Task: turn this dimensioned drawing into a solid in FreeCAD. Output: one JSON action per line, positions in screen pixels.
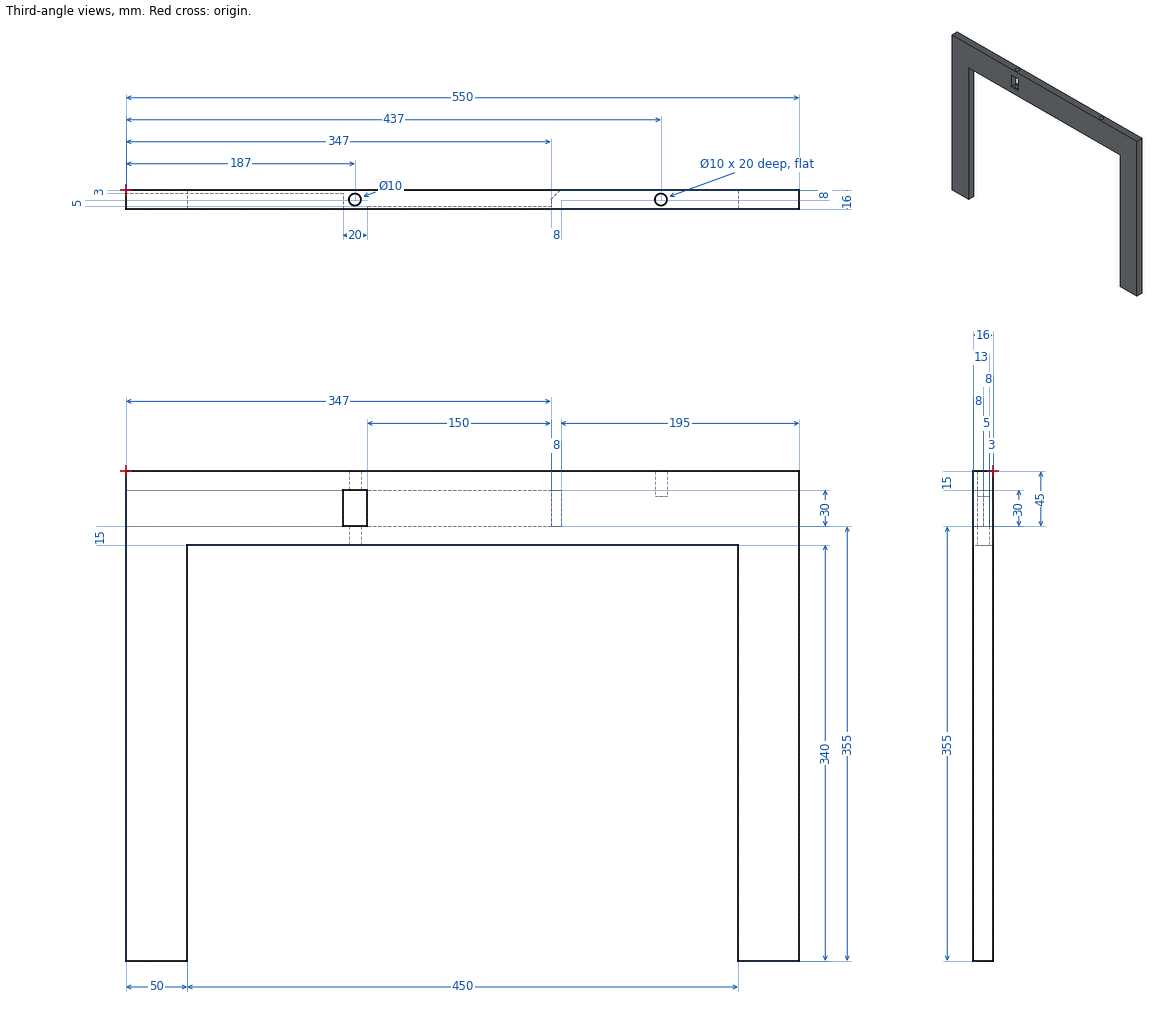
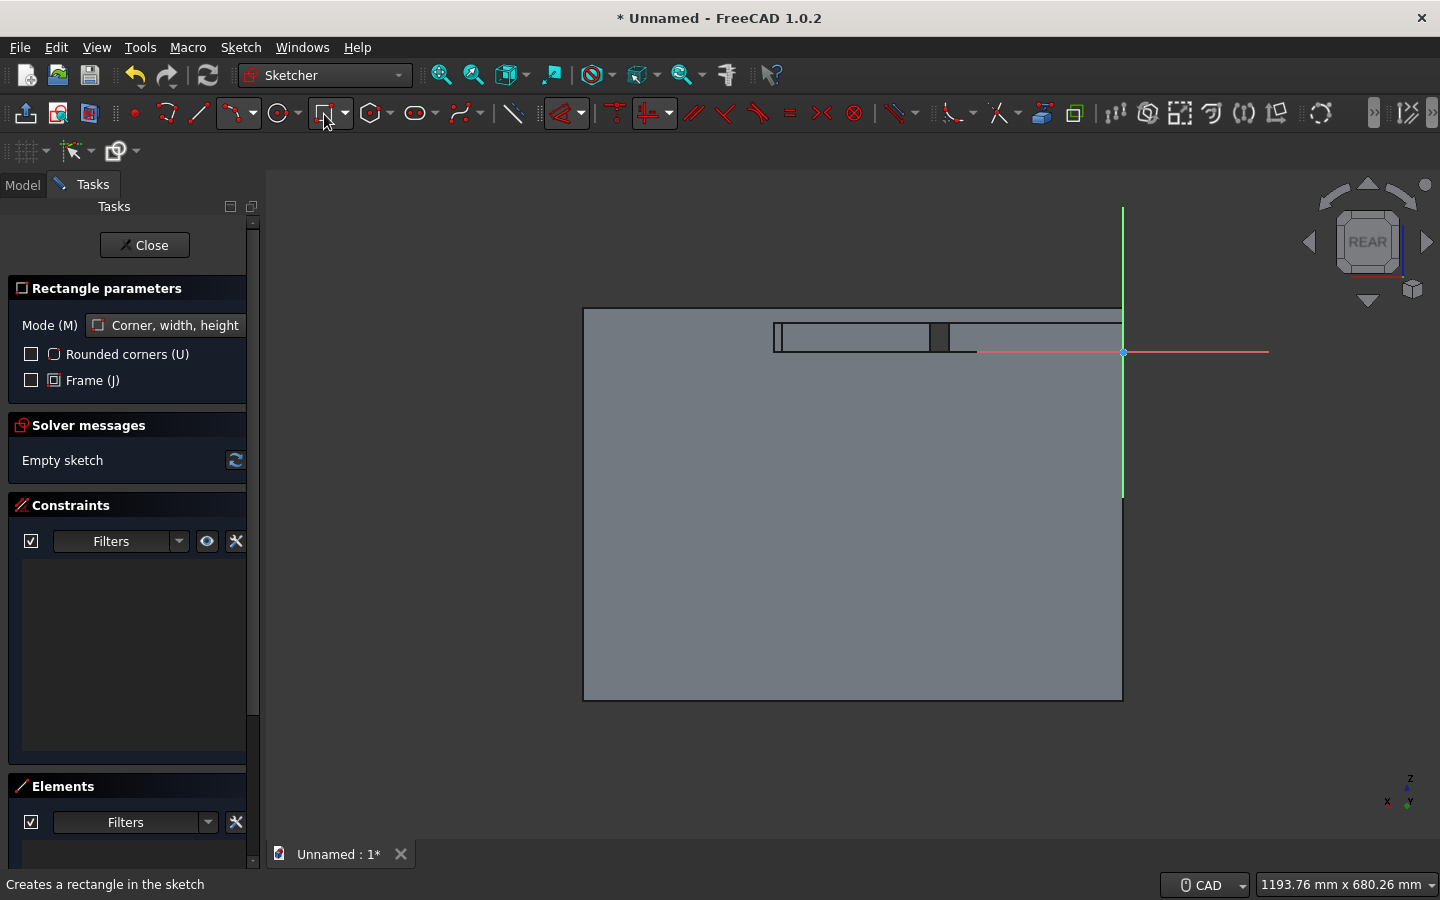
{"action": "left_click", "coordinate": [632, 367]}
{"action": "left_click", "coordinate": [1074, 701]}
{"action": "key", "text": "Escape"}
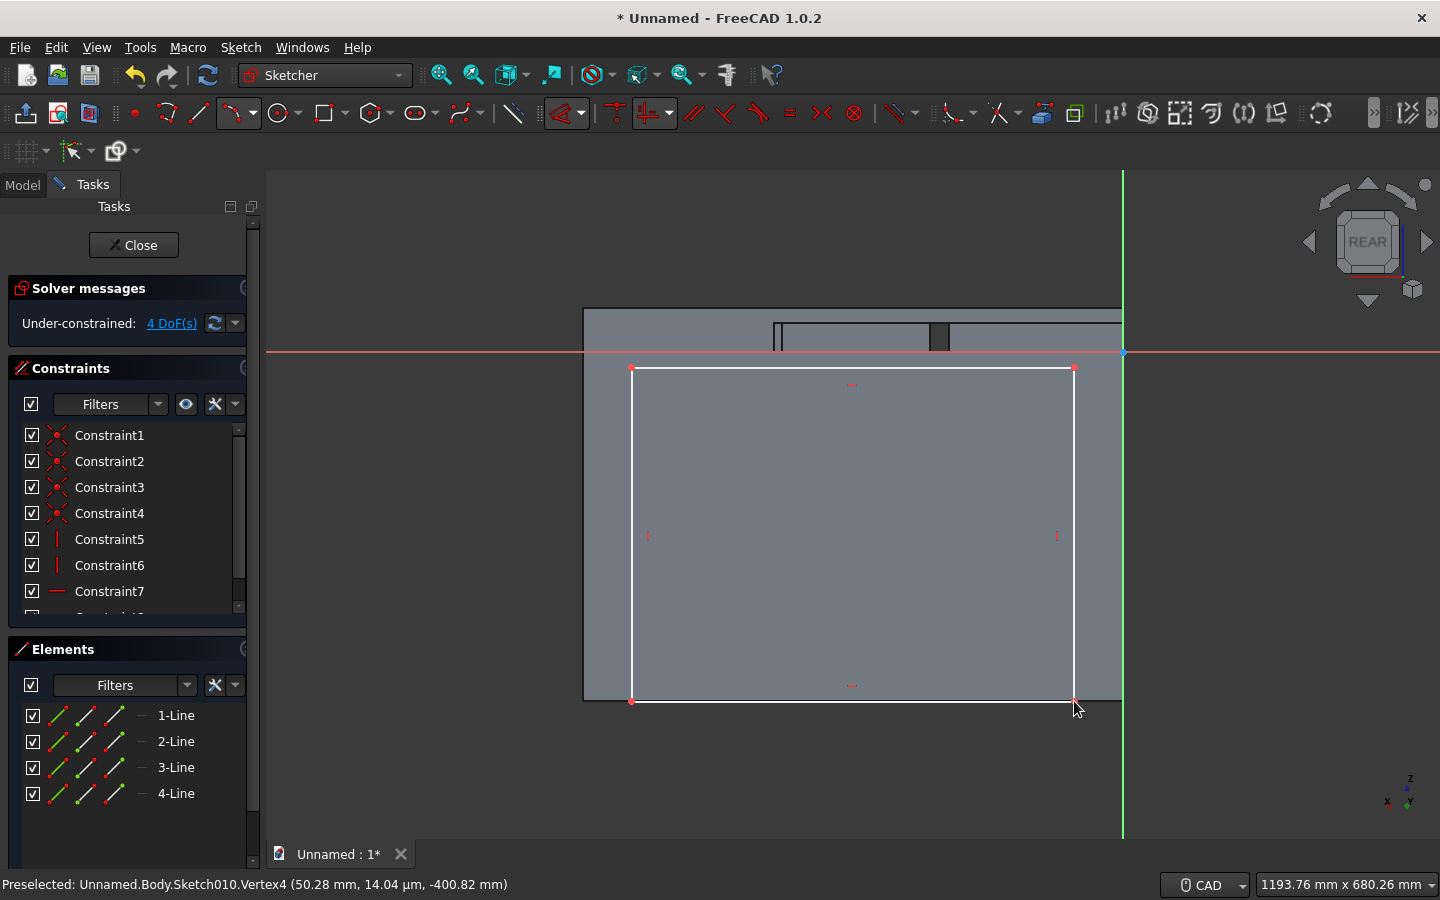
{"action": "left_click", "coordinate": [632, 468]}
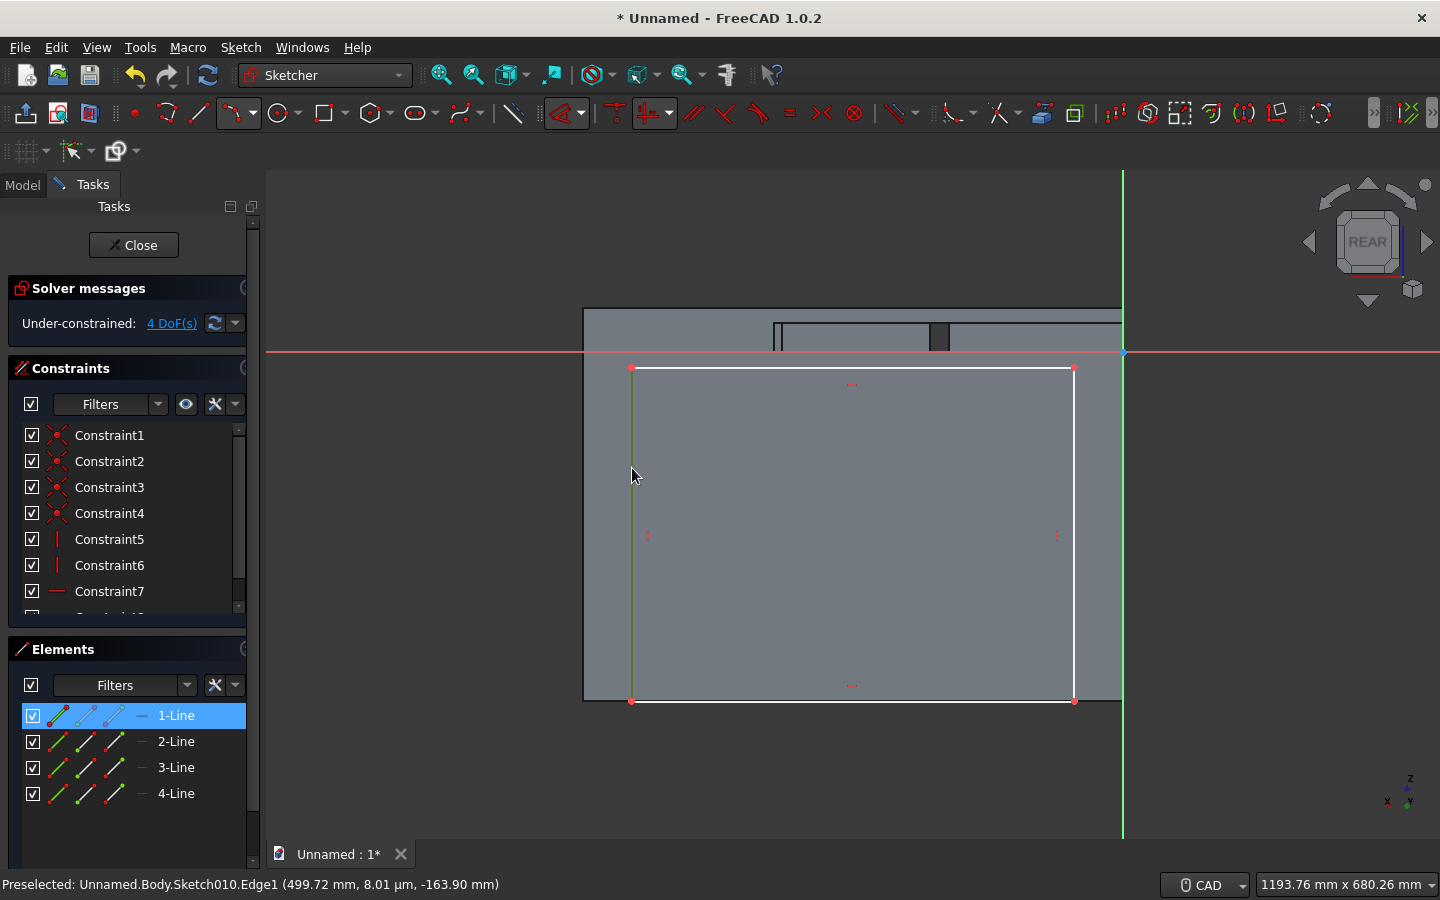
{"action": "left_click", "coordinate": [584, 114]}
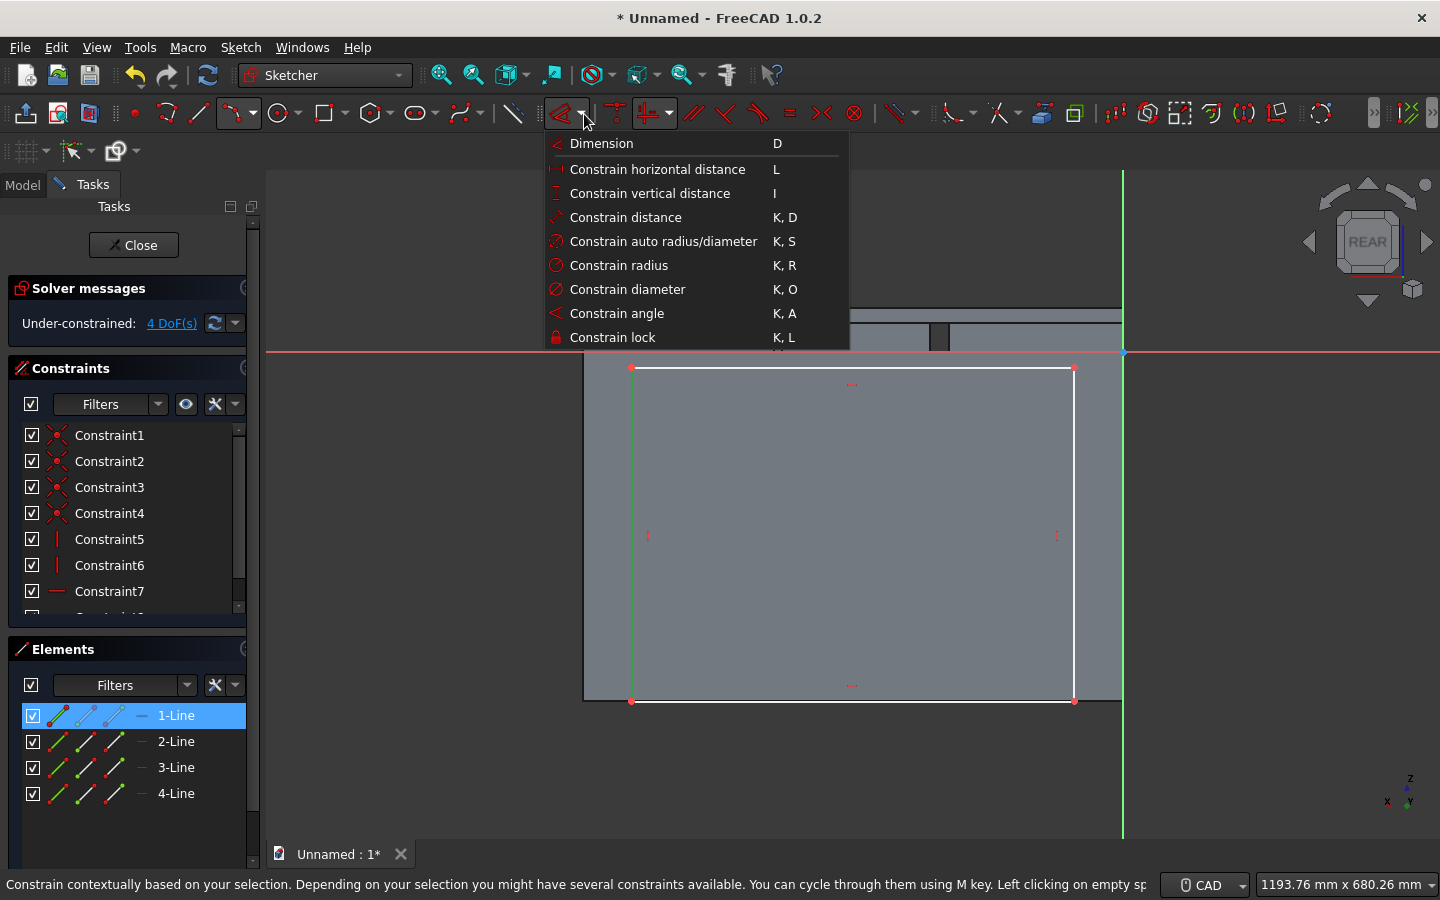
{"action": "left_click", "coordinate": [697, 193]}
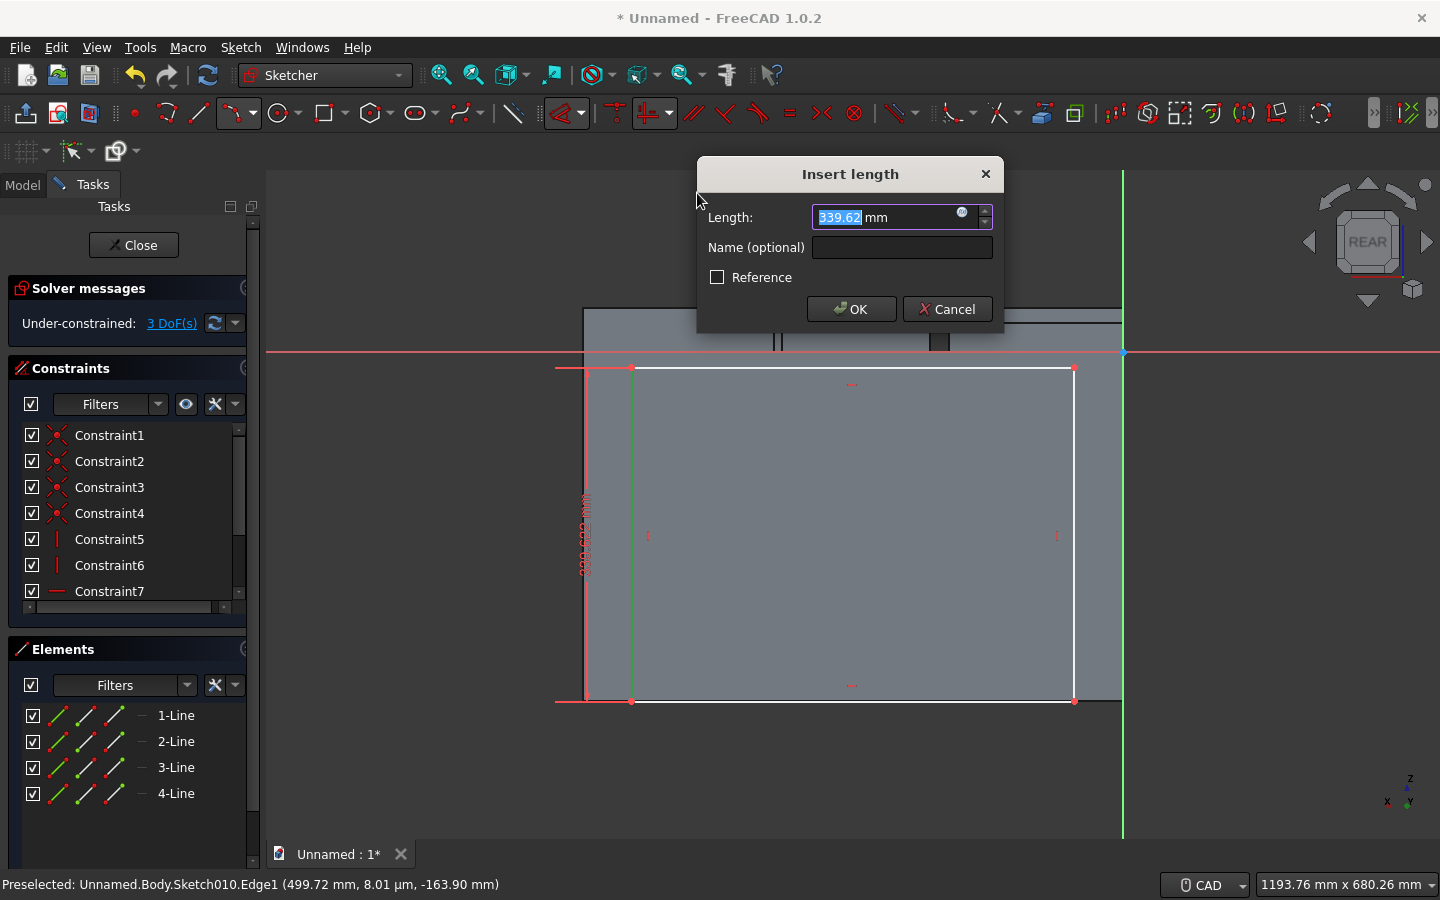
{"action": "type", "text": "340"}
{"action": "key", "text": "Return"}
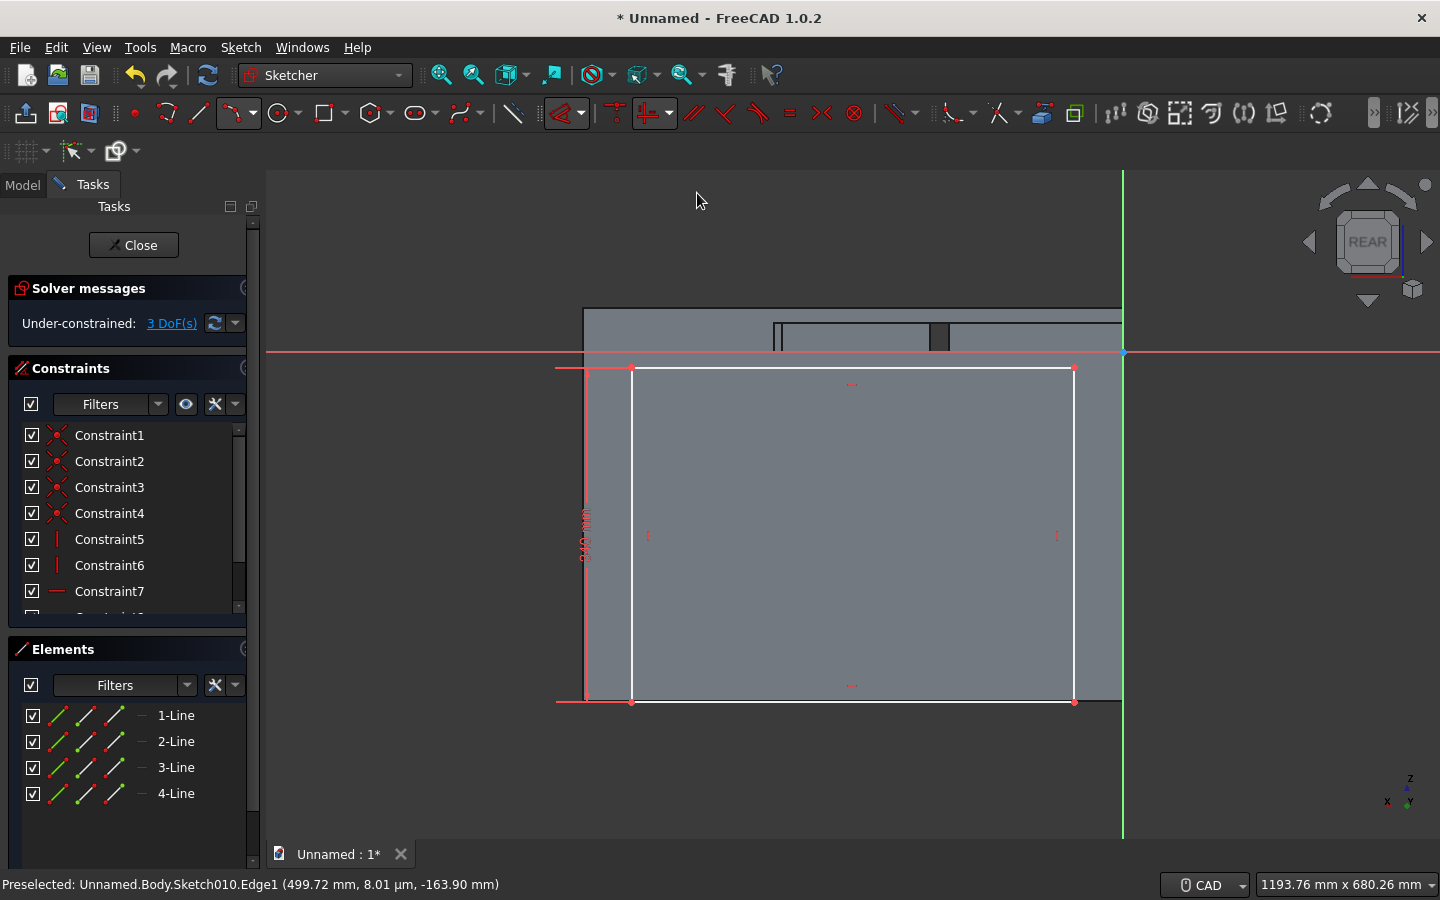
{"action": "left_click", "coordinate": [765, 702]}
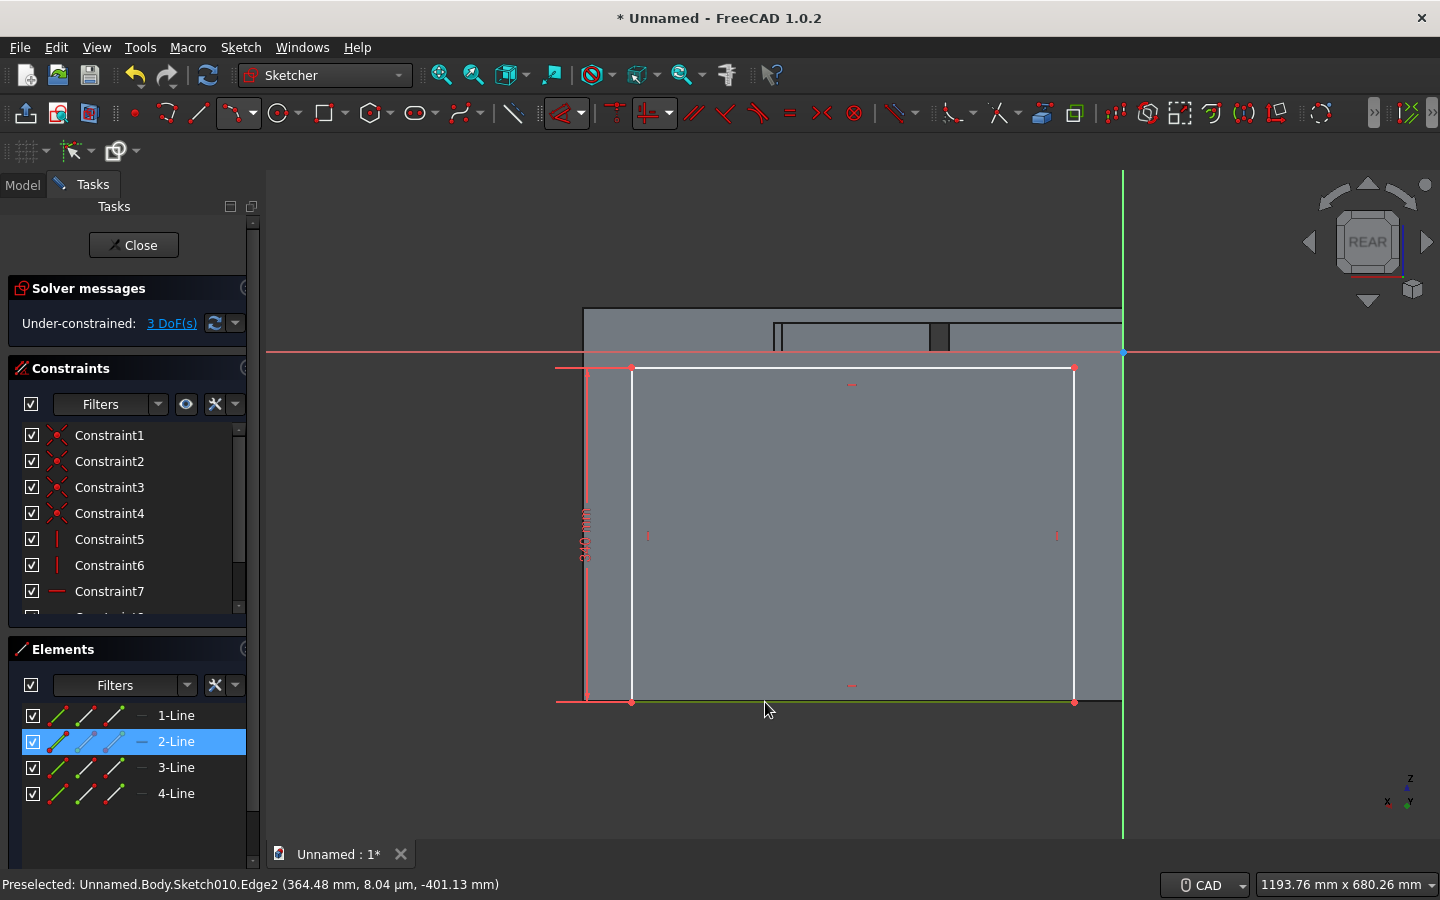
{"action": "key", "text": "l"}